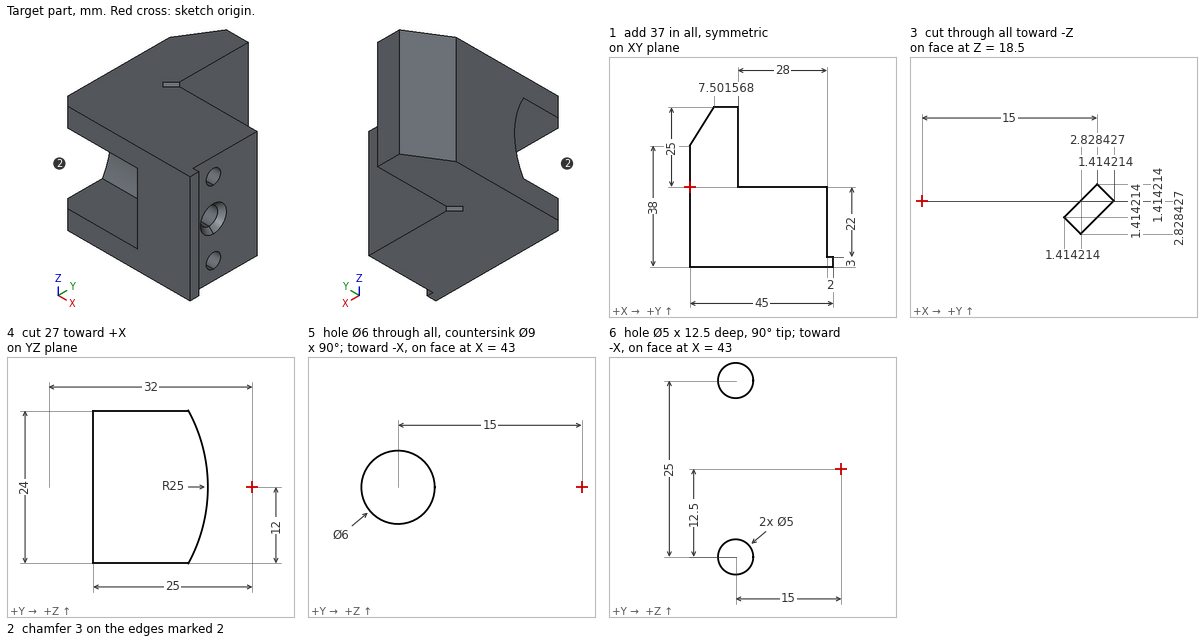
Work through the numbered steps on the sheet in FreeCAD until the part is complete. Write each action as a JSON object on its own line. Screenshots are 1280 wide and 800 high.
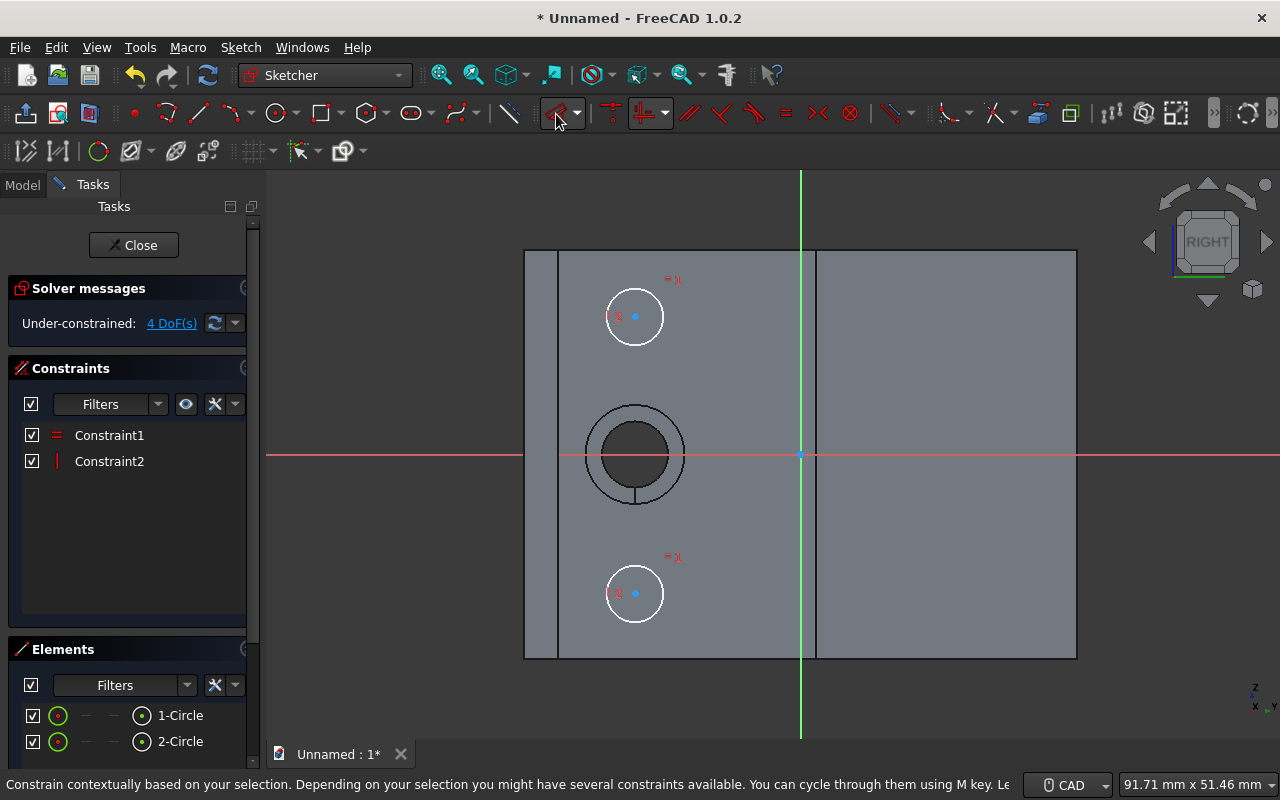
{"action": "left_click", "coordinate": [655, 574]}
{"action": "left_click", "coordinate": [678, 551]}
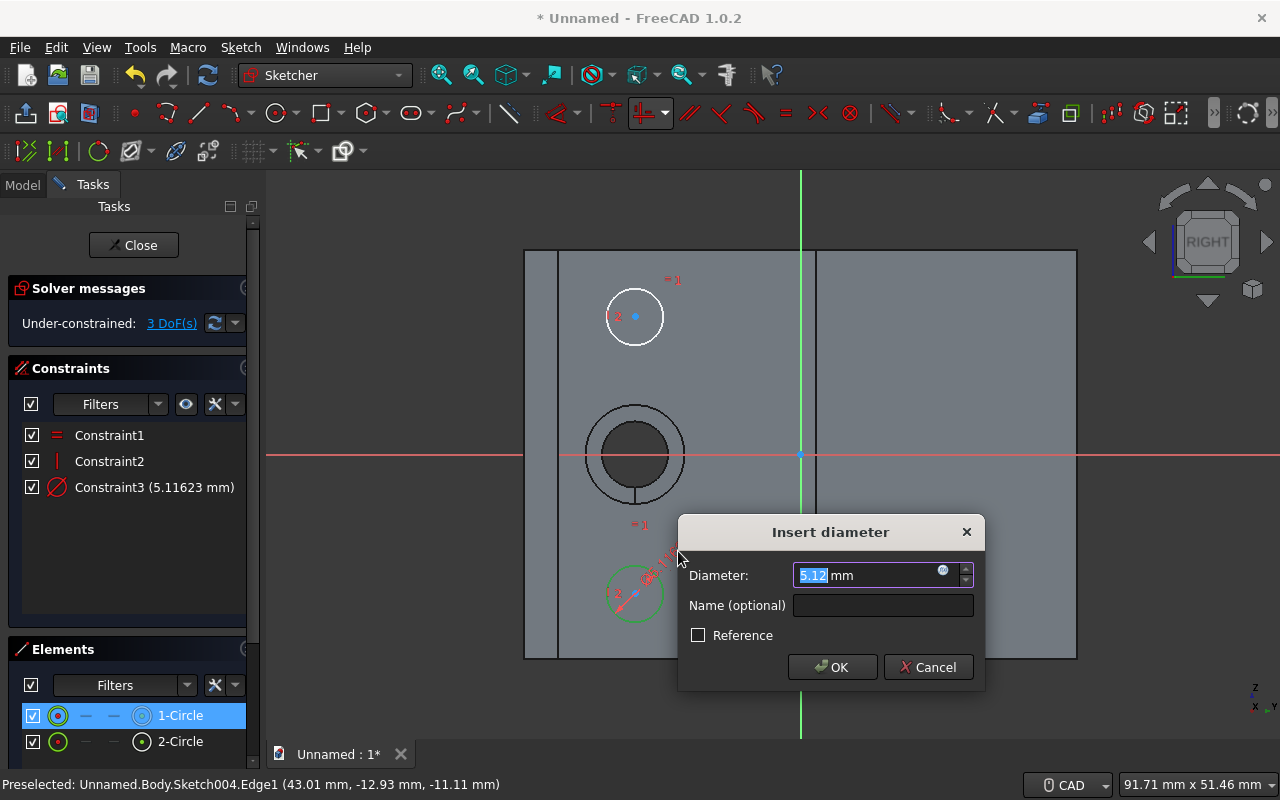
{"action": "type", "text": "5"}
{"action": "key", "text": "Return"}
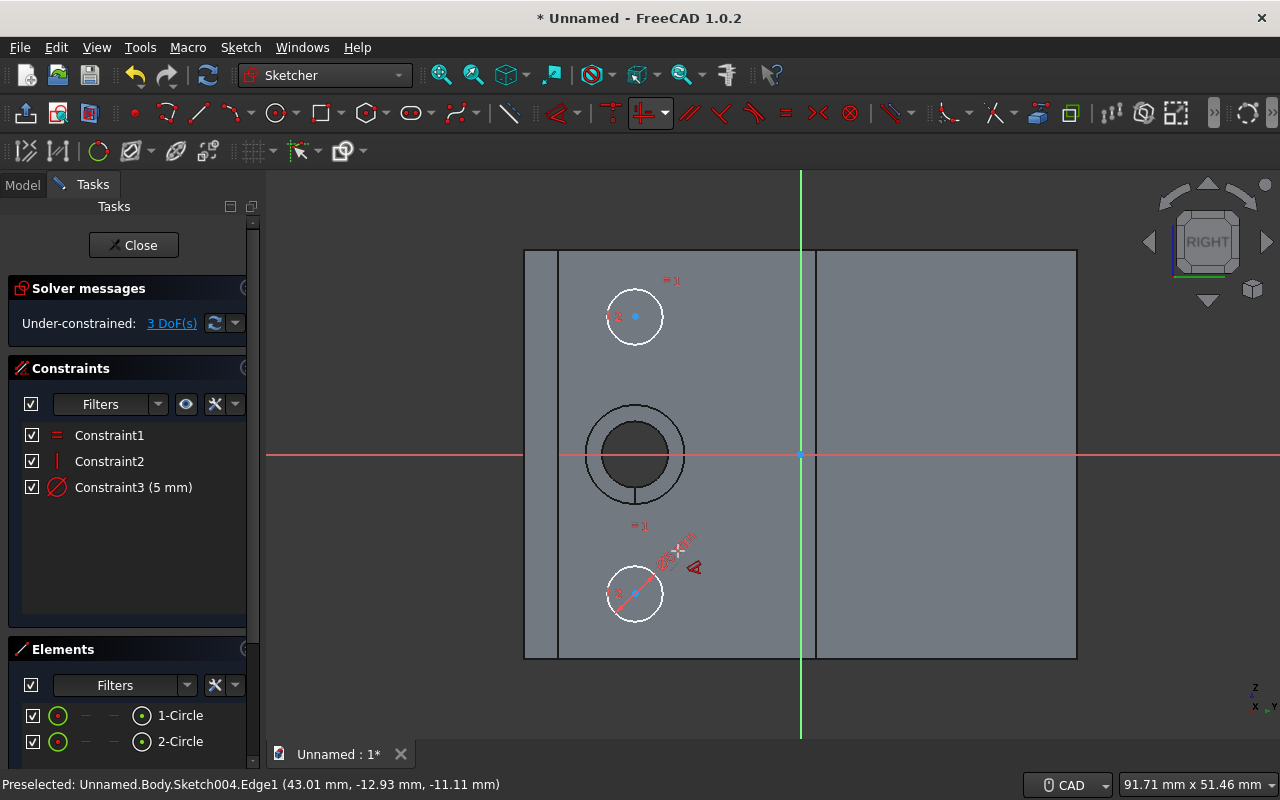
{"action": "left_click", "coordinate": [635, 594]}
{"action": "left_click", "coordinate": [718, 628]}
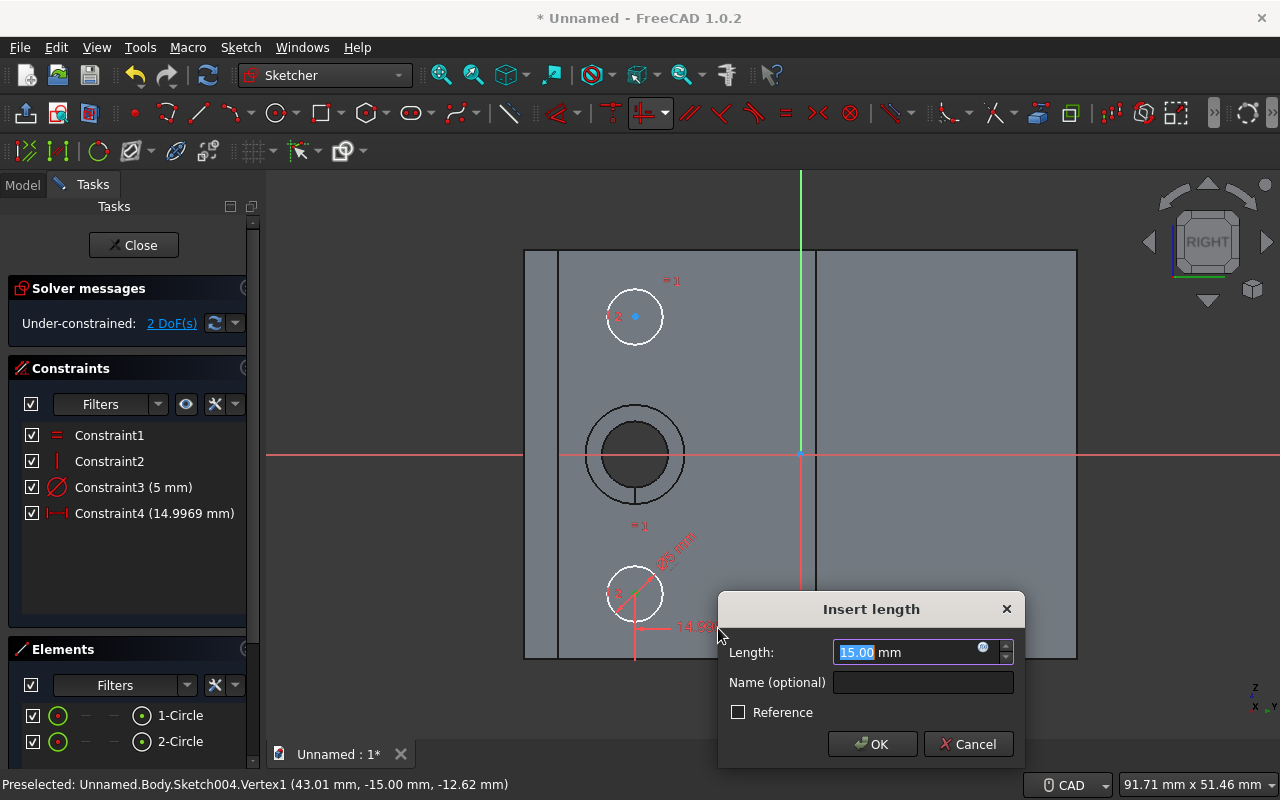
{"action": "type", "text": "15"}
{"action": "key", "text": "Return"}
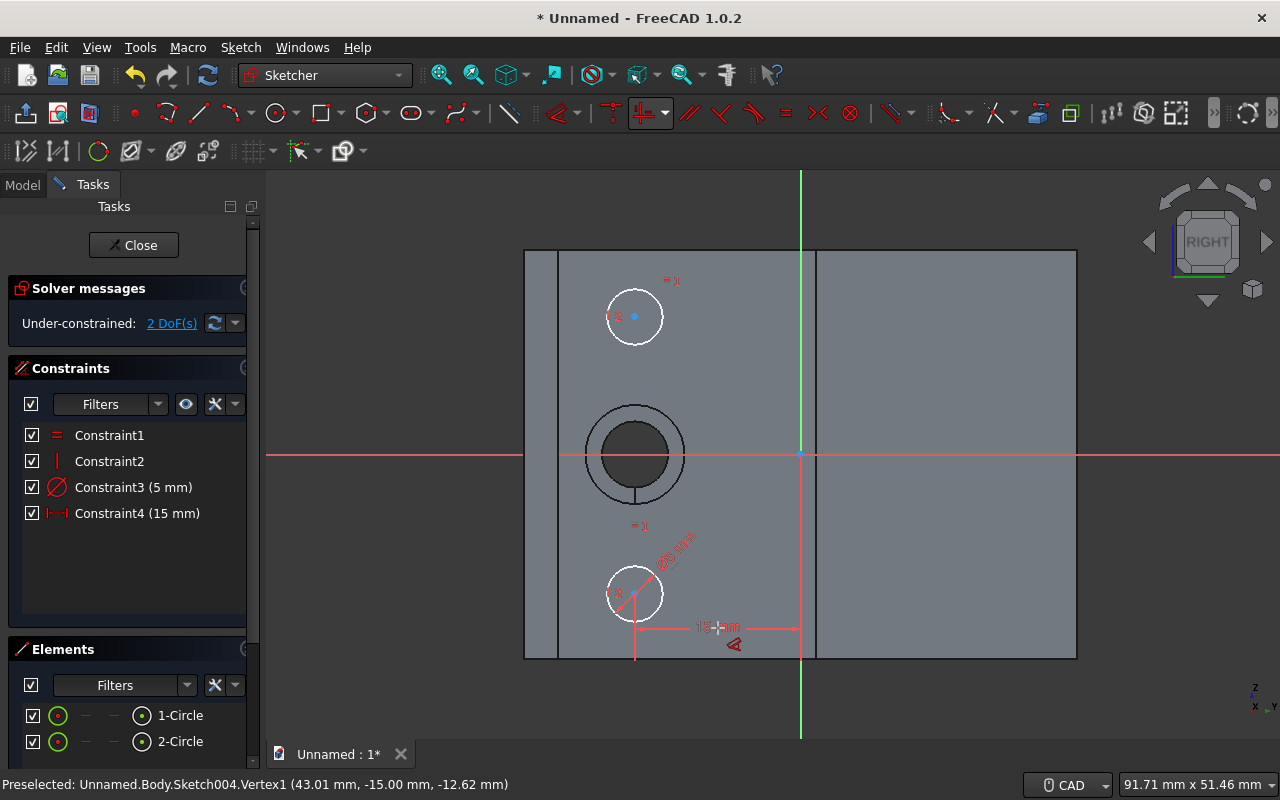
{"action": "left_click", "coordinate": [635, 594]}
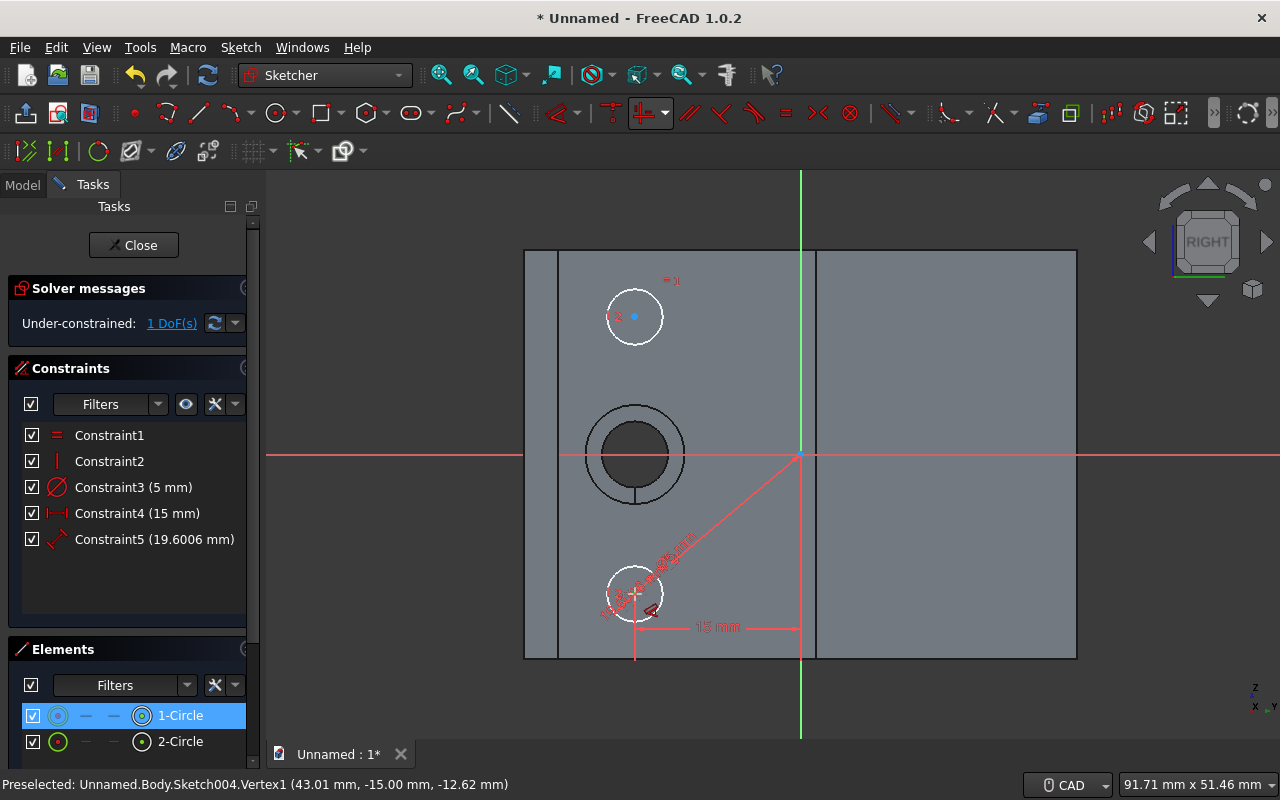
{"action": "left_click", "coordinate": [635, 317]}
{"action": "left_click", "coordinate": [601, 392]}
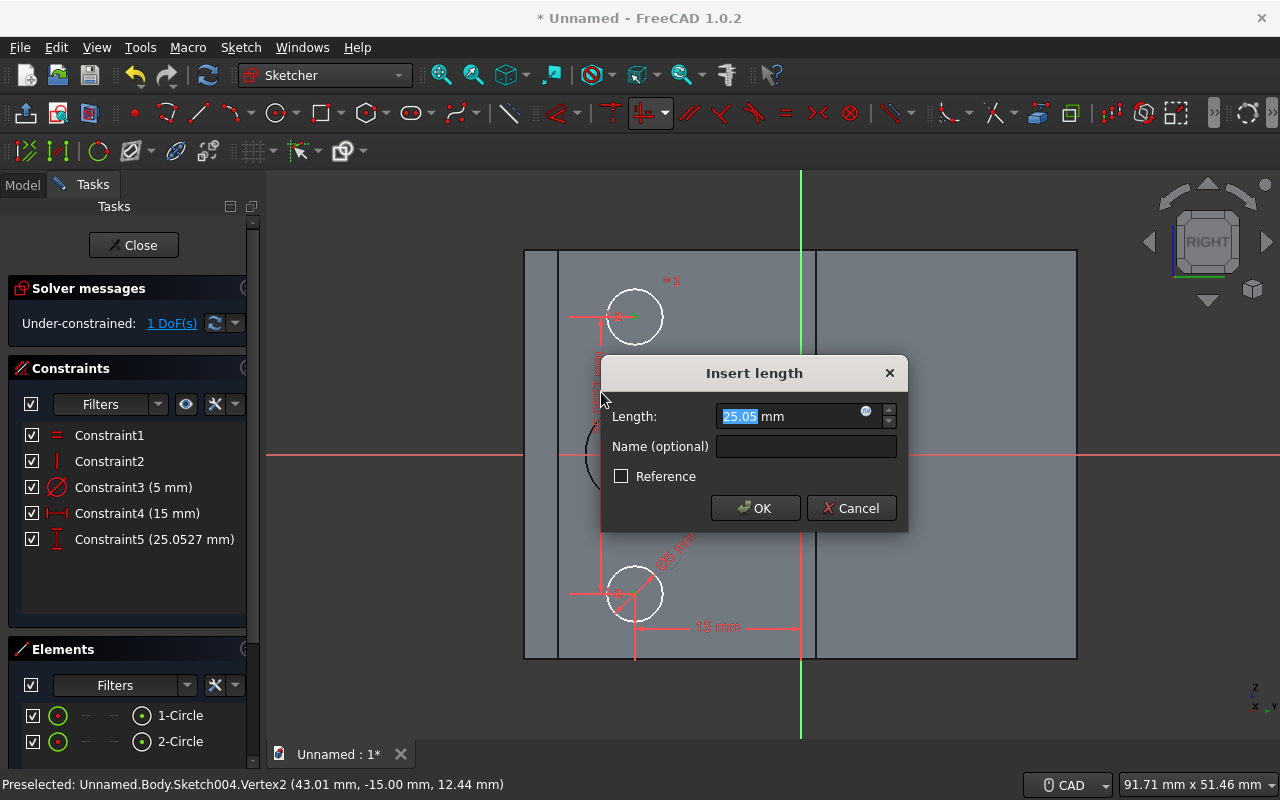
{"action": "type", "text": "25"}
{"action": "key", "text": "Return"}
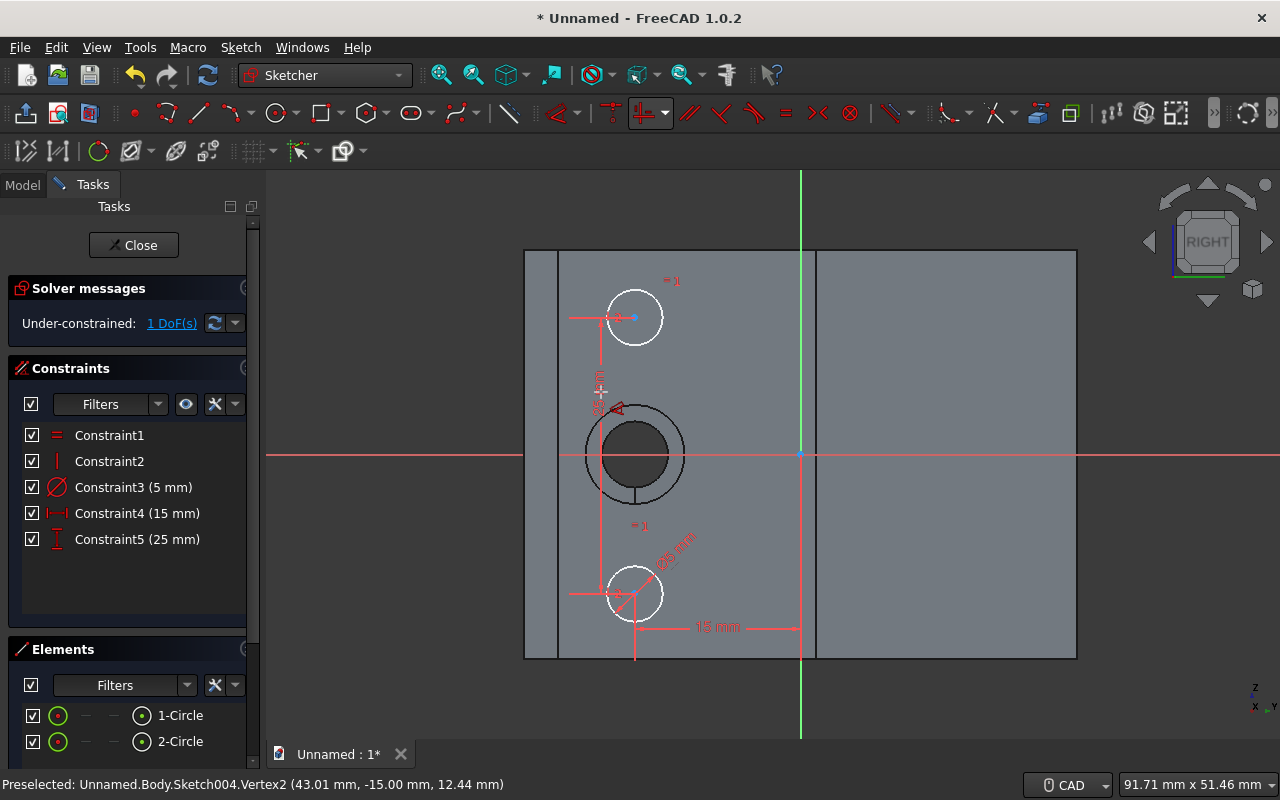
{"action": "left_click", "coordinate": [635, 594]}
{"action": "left_click", "coordinate": [835, 524]}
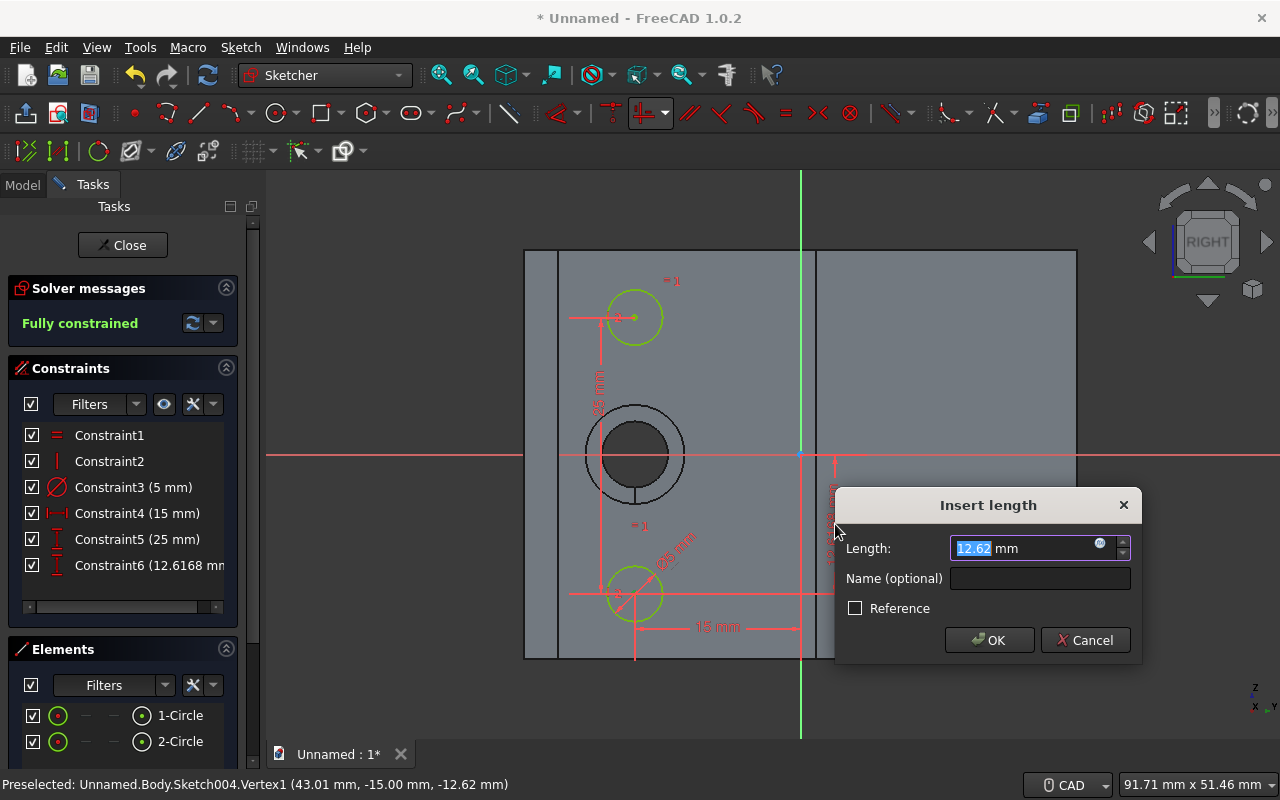
{"action": "type", "text": "12.5"}
{"action": "key", "text": "Return"}
{"action": "key", "text": "Escape"}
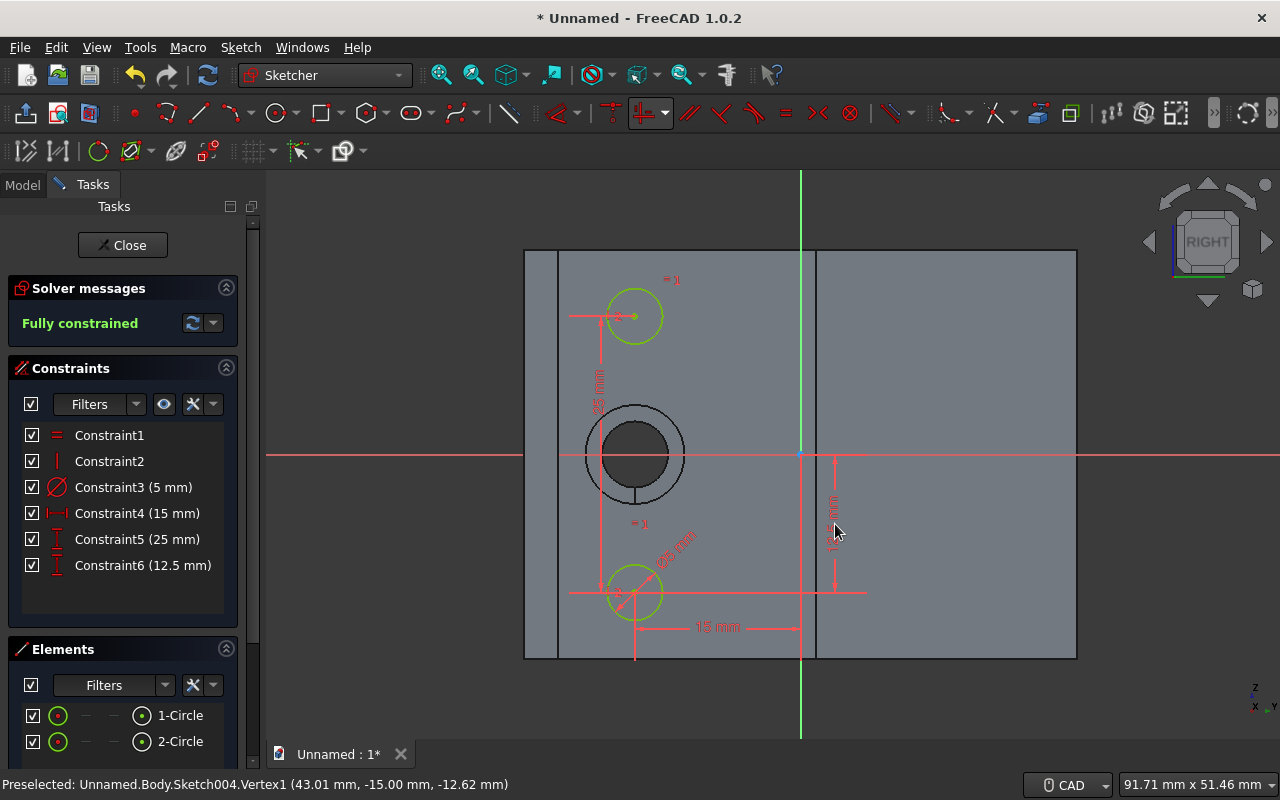
{"action": "left_click", "coordinate": [123, 245]}